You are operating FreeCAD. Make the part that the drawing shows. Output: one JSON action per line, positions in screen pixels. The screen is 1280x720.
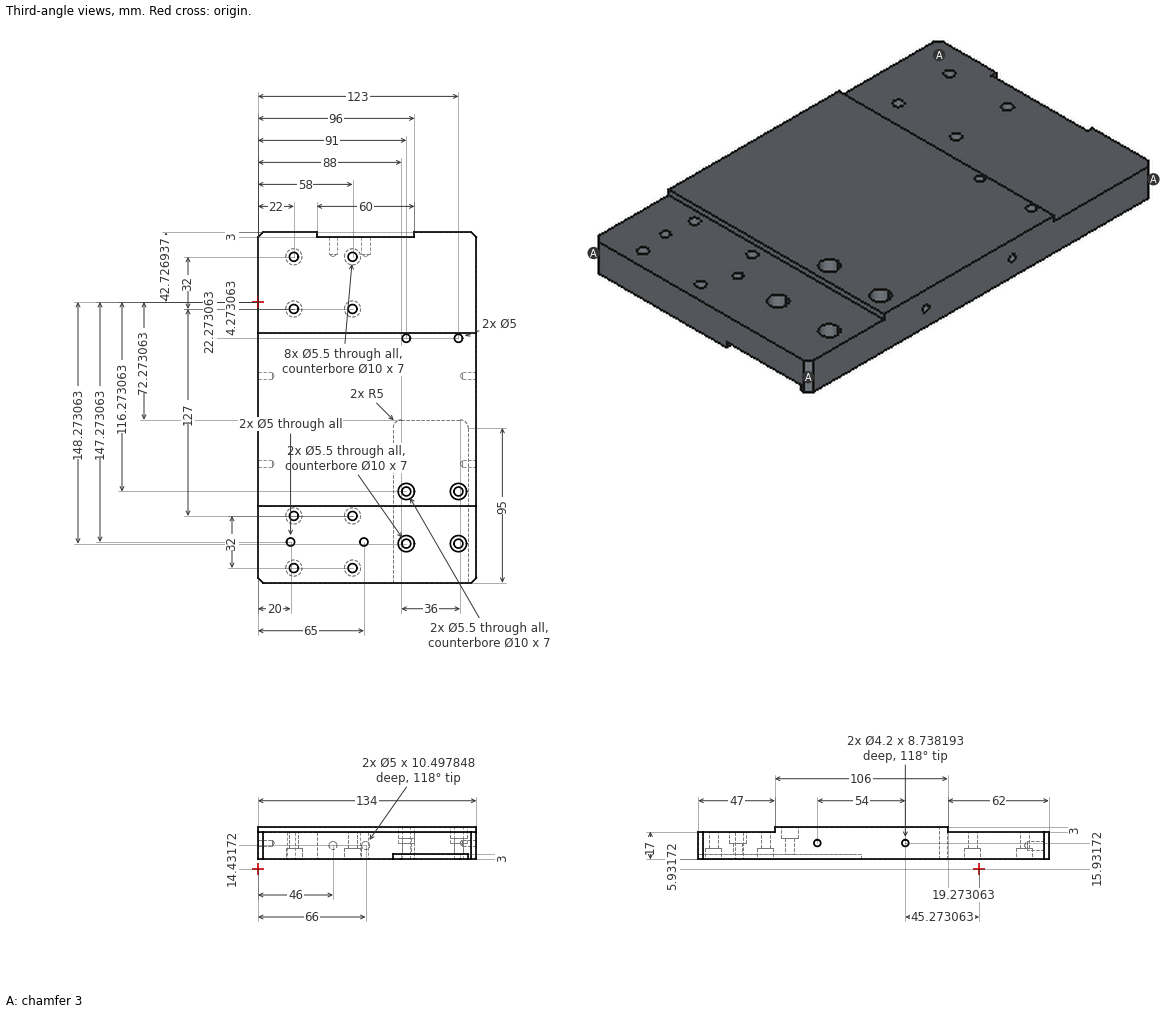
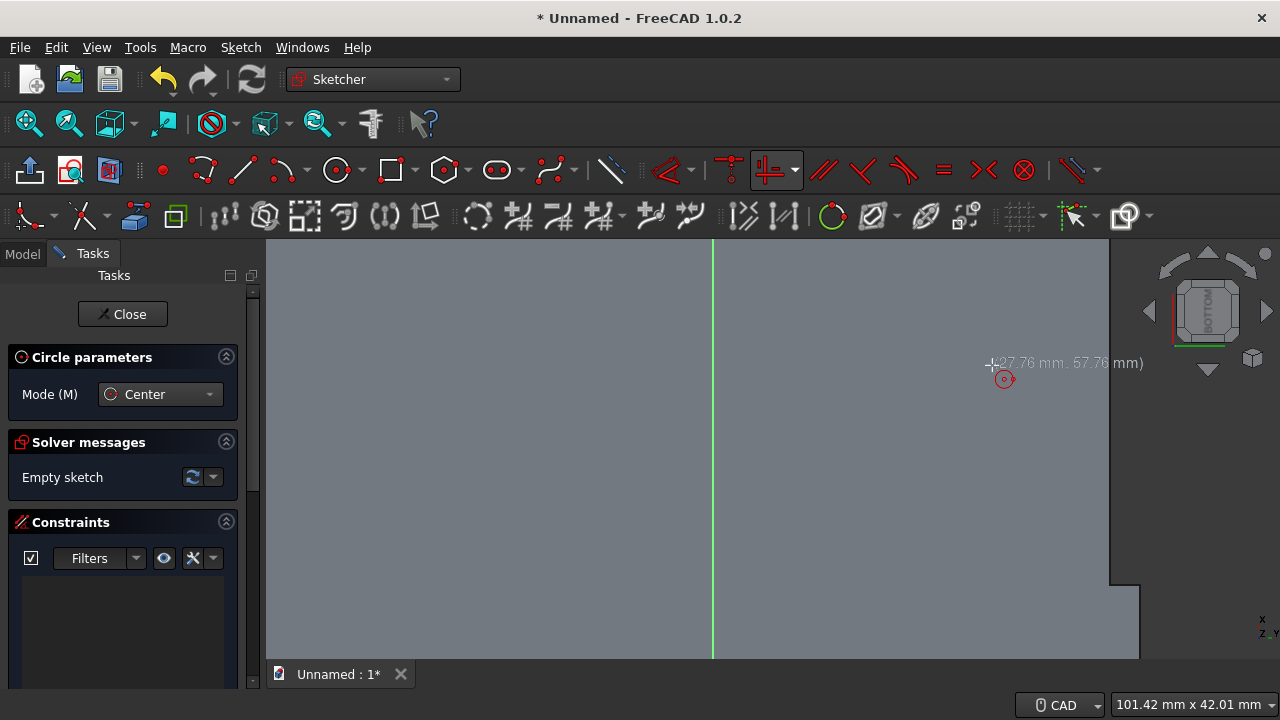
{"action": "left_click", "coordinate": [990, 365]}
{"action": "mouse_move", "coordinate": [1009, 346]}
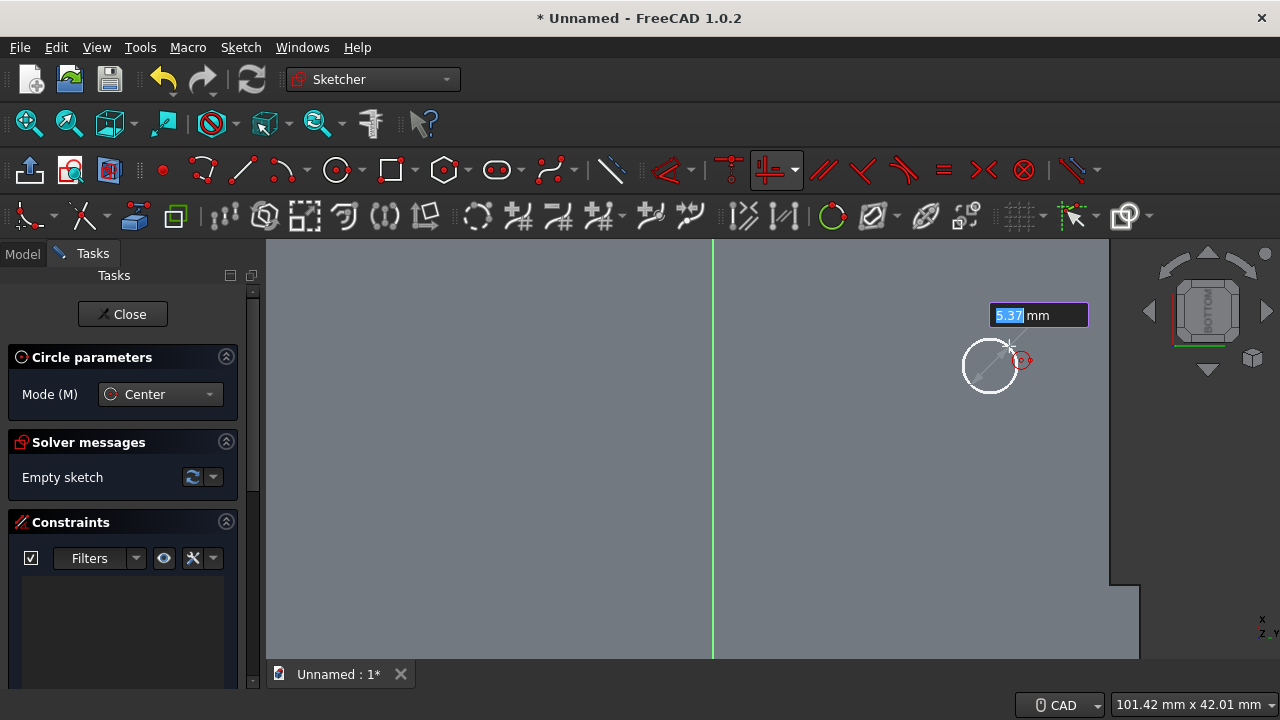
{"action": "type", "text": "5.5"}
{"action": "key", "text": "Return"}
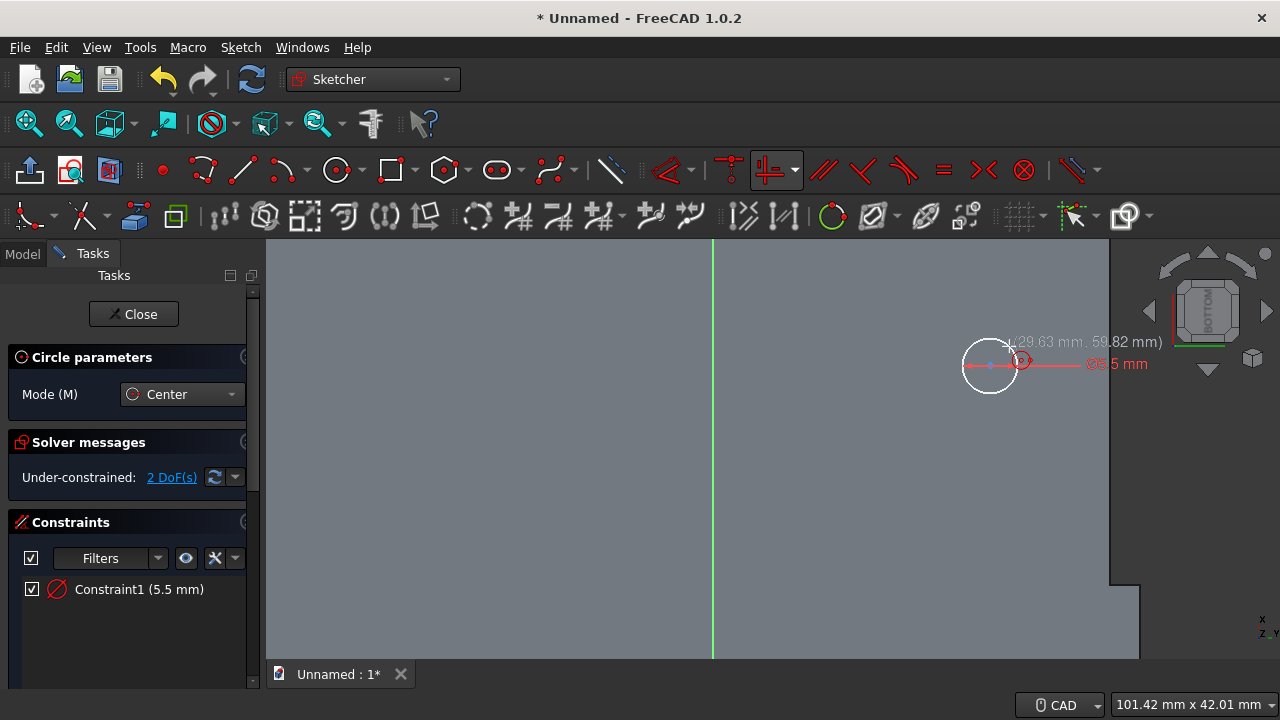
{"action": "scroll", "coordinate": [993, 366], "scroll_direction": "down", "scroll_amount": 6}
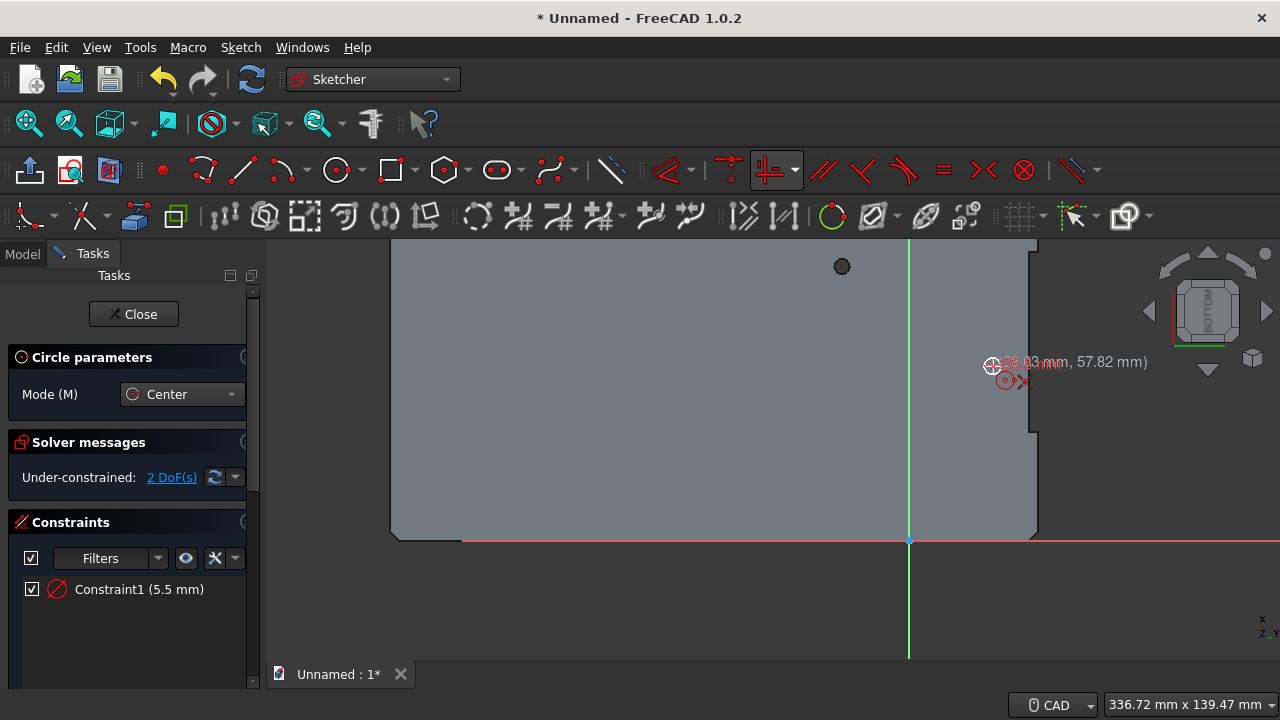
{"action": "scroll", "coordinate": [993, 474], "scroll_direction": "up", "scroll_amount": 6}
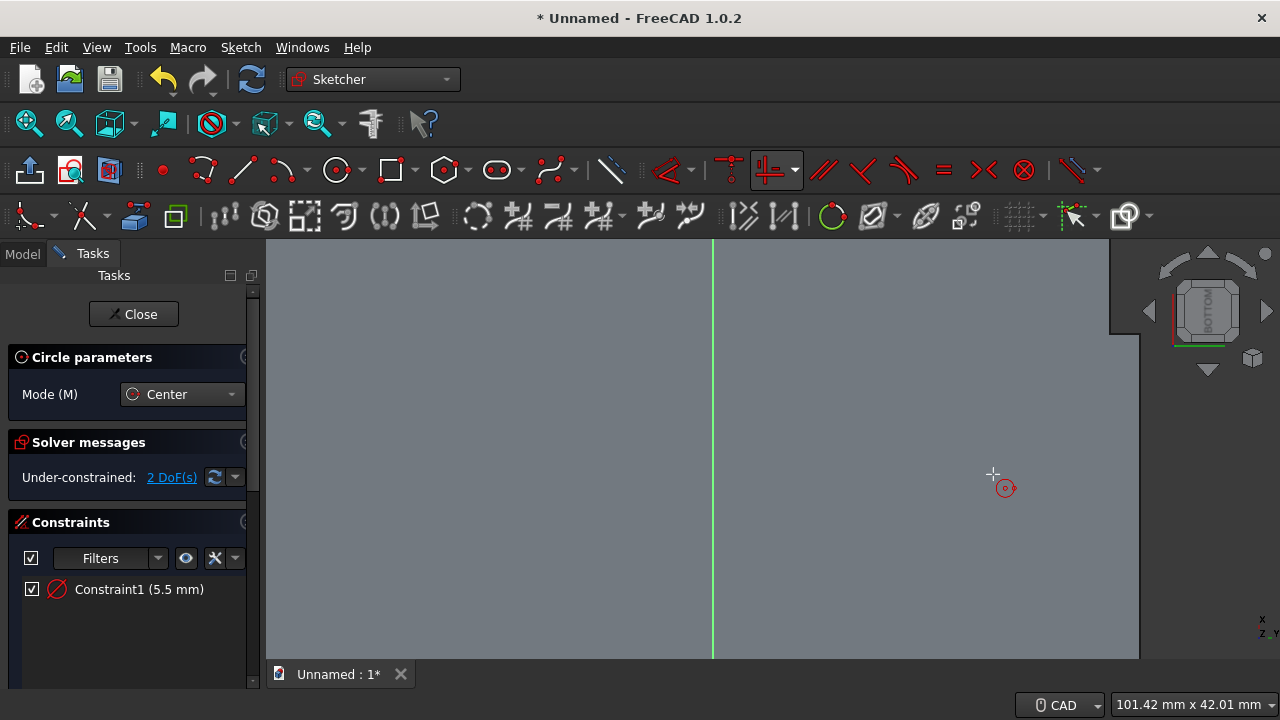
{"action": "left_click", "coordinate": [990, 474]}
{"action": "mouse_move", "coordinate": [1009, 455]}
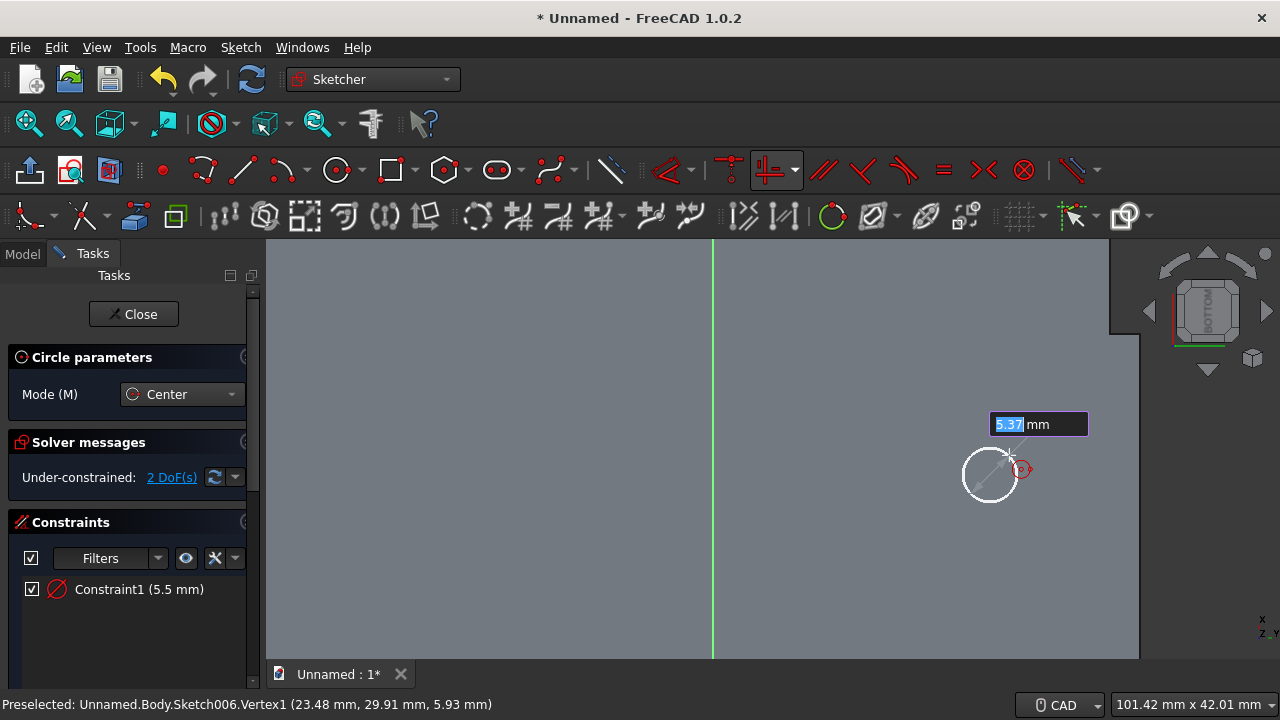
{"action": "type", "text": "5.5"}
{"action": "key", "text": "Return"}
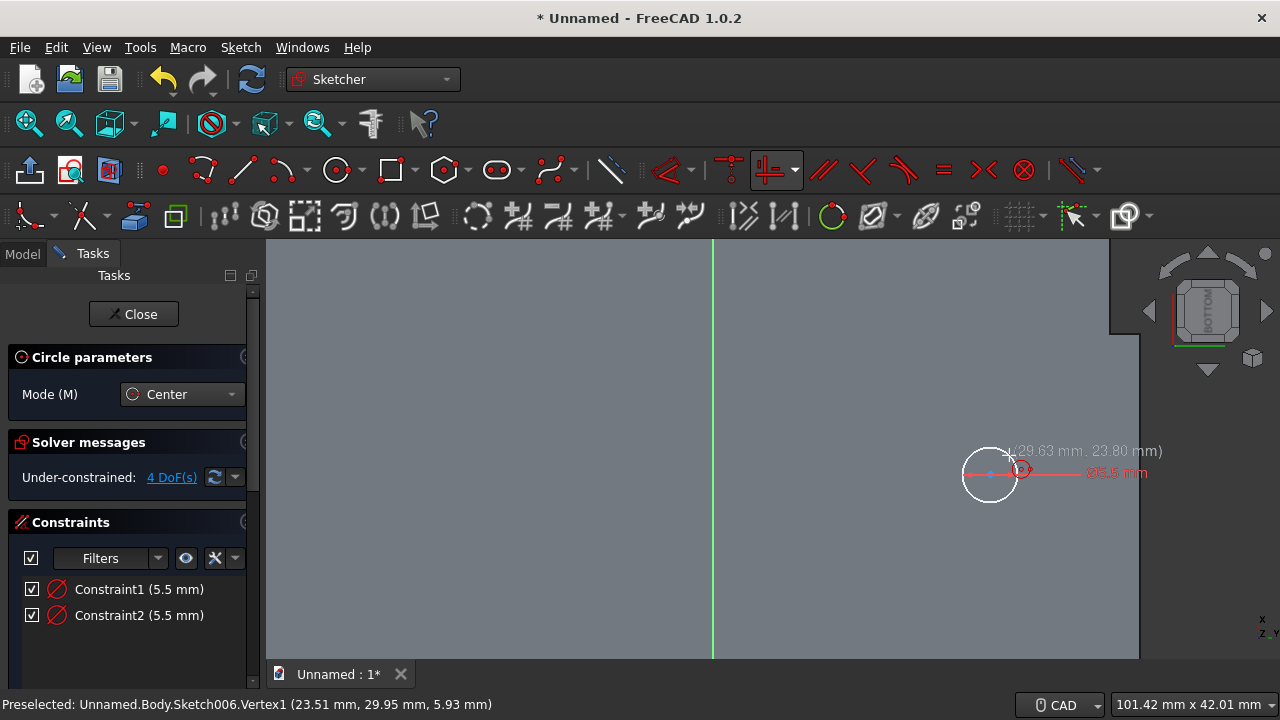
{"action": "left_click", "coordinate": [670, 474]}
{"action": "mouse_move", "coordinate": [689, 455]}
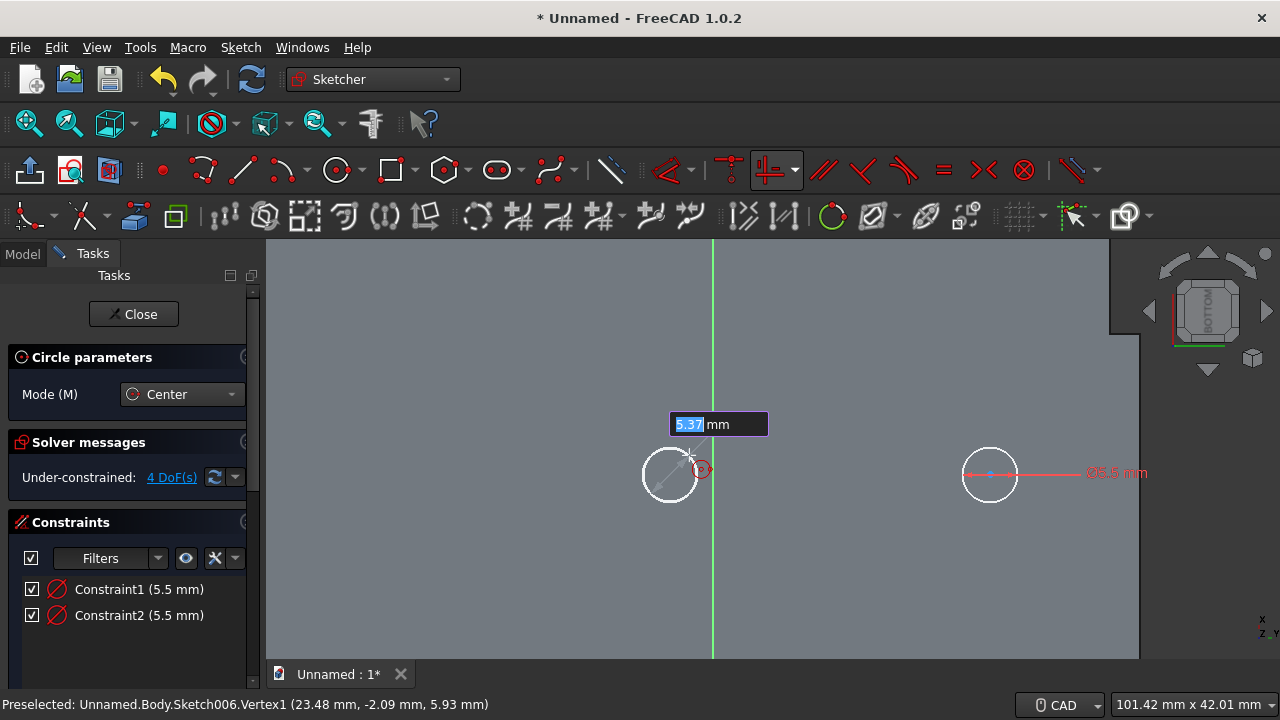
{"action": "type", "text": "5.5"}
{"action": "key", "text": "Return"}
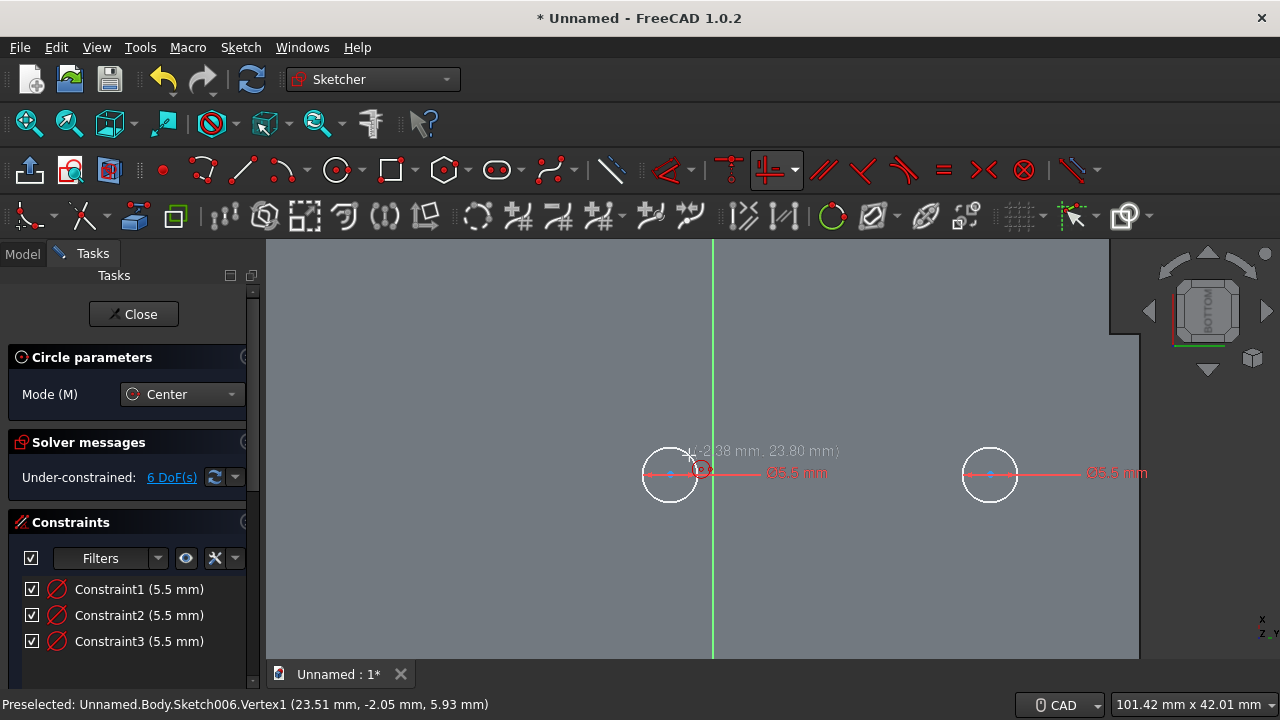
{"action": "scroll", "coordinate": [993, 474], "scroll_direction": "down", "scroll_amount": 6}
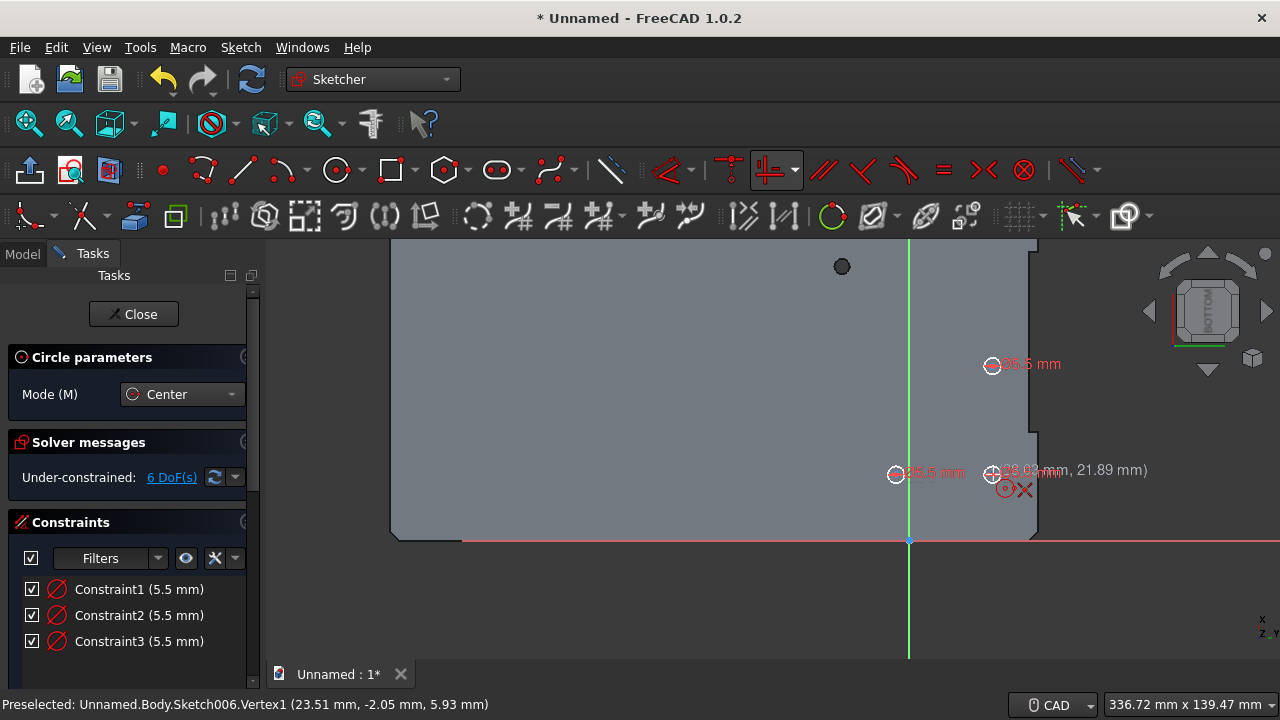
{"action": "scroll", "coordinate": [896, 366], "scroll_direction": "up", "scroll_amount": 6}